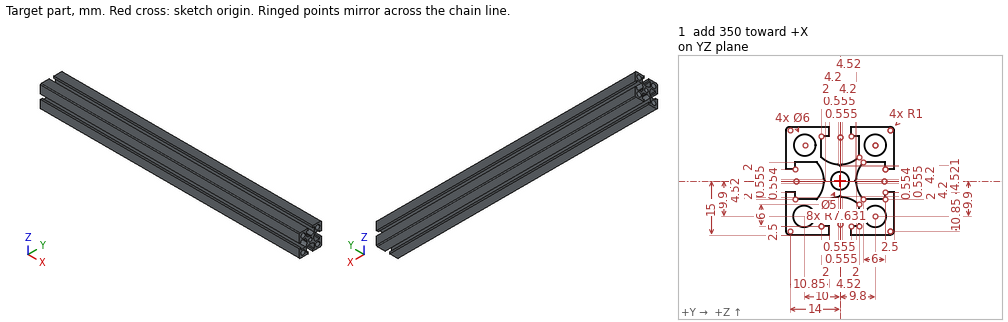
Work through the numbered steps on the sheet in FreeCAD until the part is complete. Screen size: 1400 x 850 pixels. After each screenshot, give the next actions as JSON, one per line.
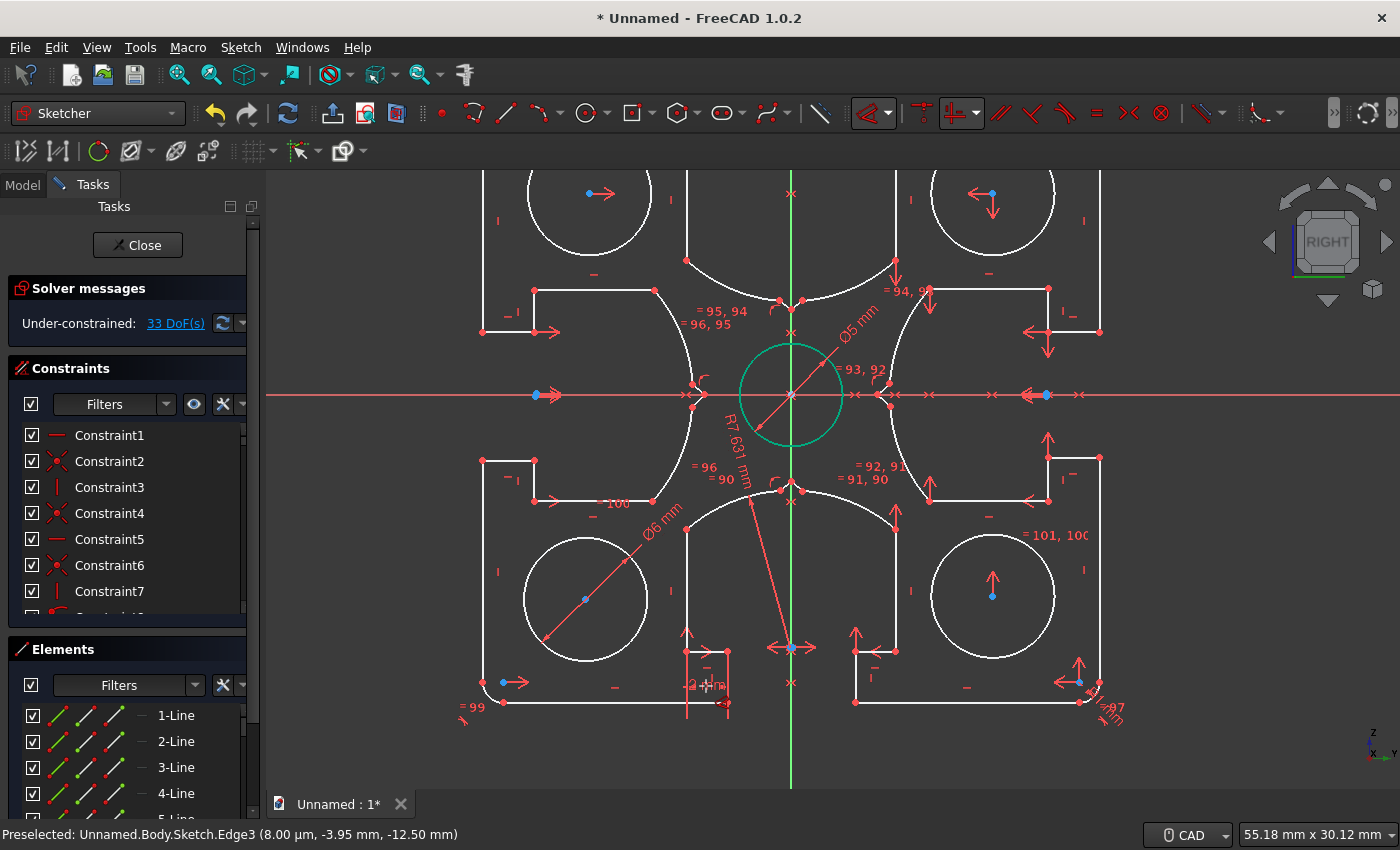
{"action": "left_click", "coordinate": [687, 615]}
{"action": "left_click", "coordinate": [653, 563]}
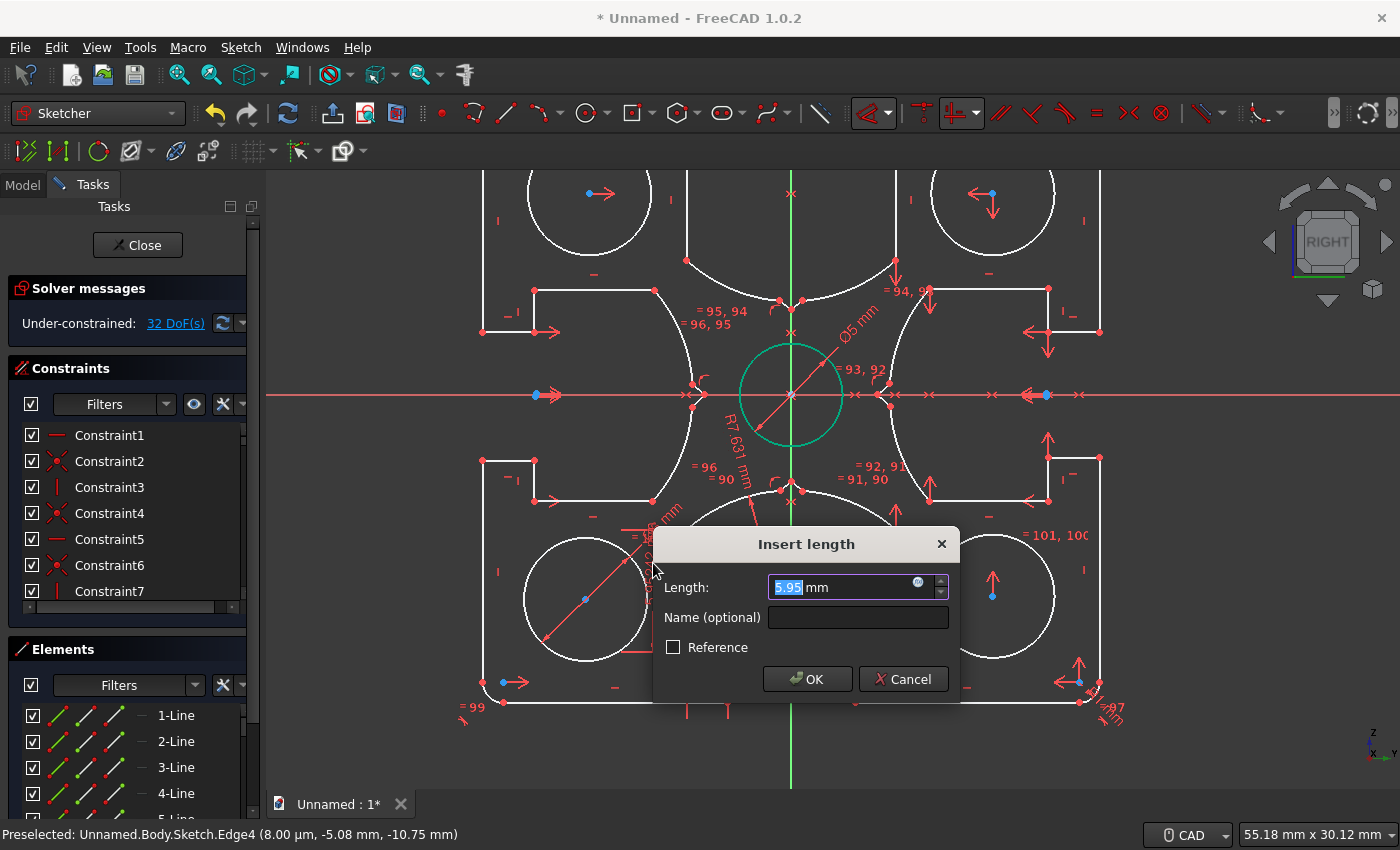
{"action": "type", "text": "6"}
{"action": "key", "text": "Return"}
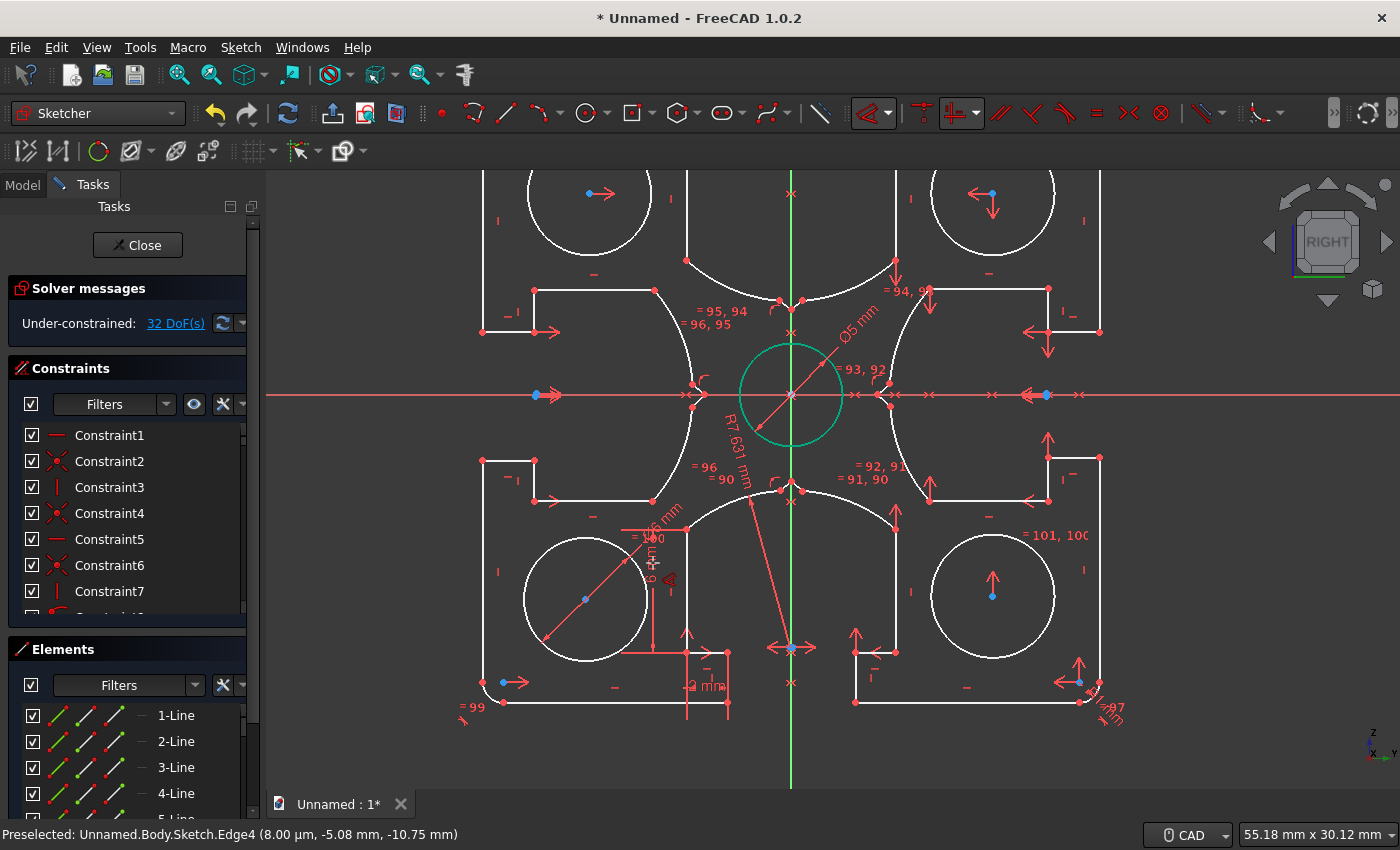
{"action": "left_click", "coordinate": [884, 653]}
{"action": "left_click", "coordinate": [876, 687]}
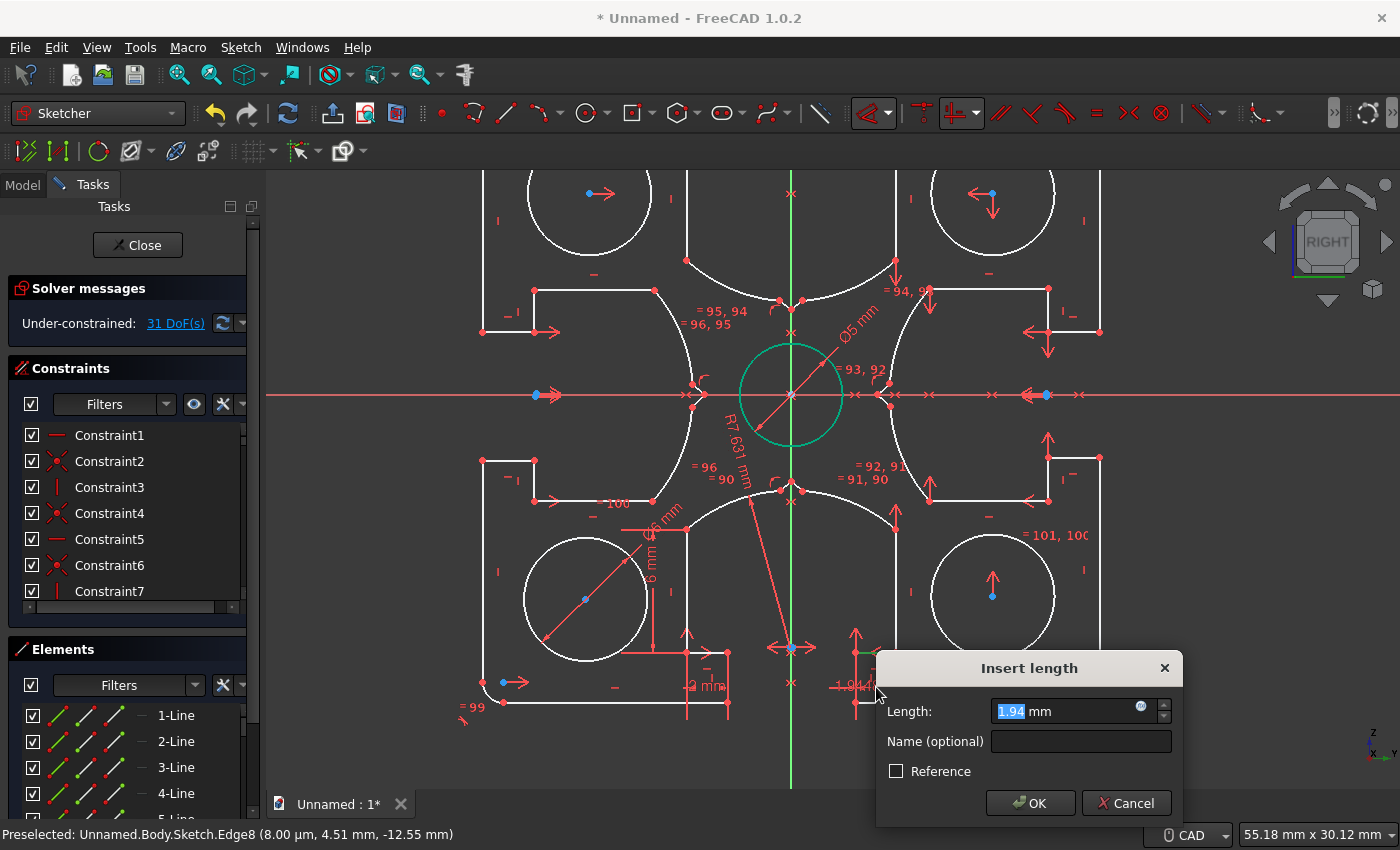
{"action": "type", "text": "2"}
{"action": "key", "text": "Return"}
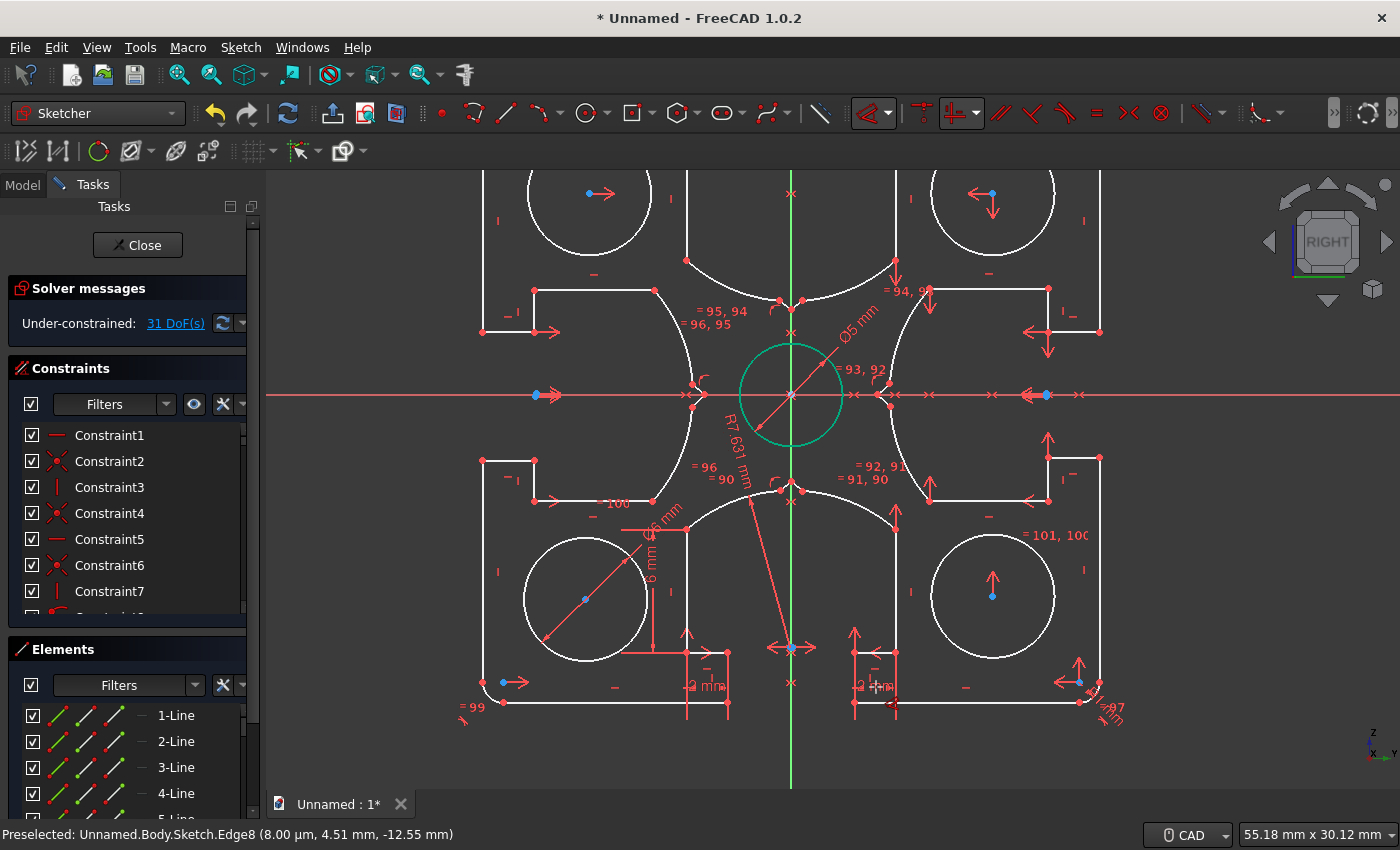
{"action": "left_click", "coordinate": [1048, 471]}
{"action": "left_click", "coordinate": [1082, 479]}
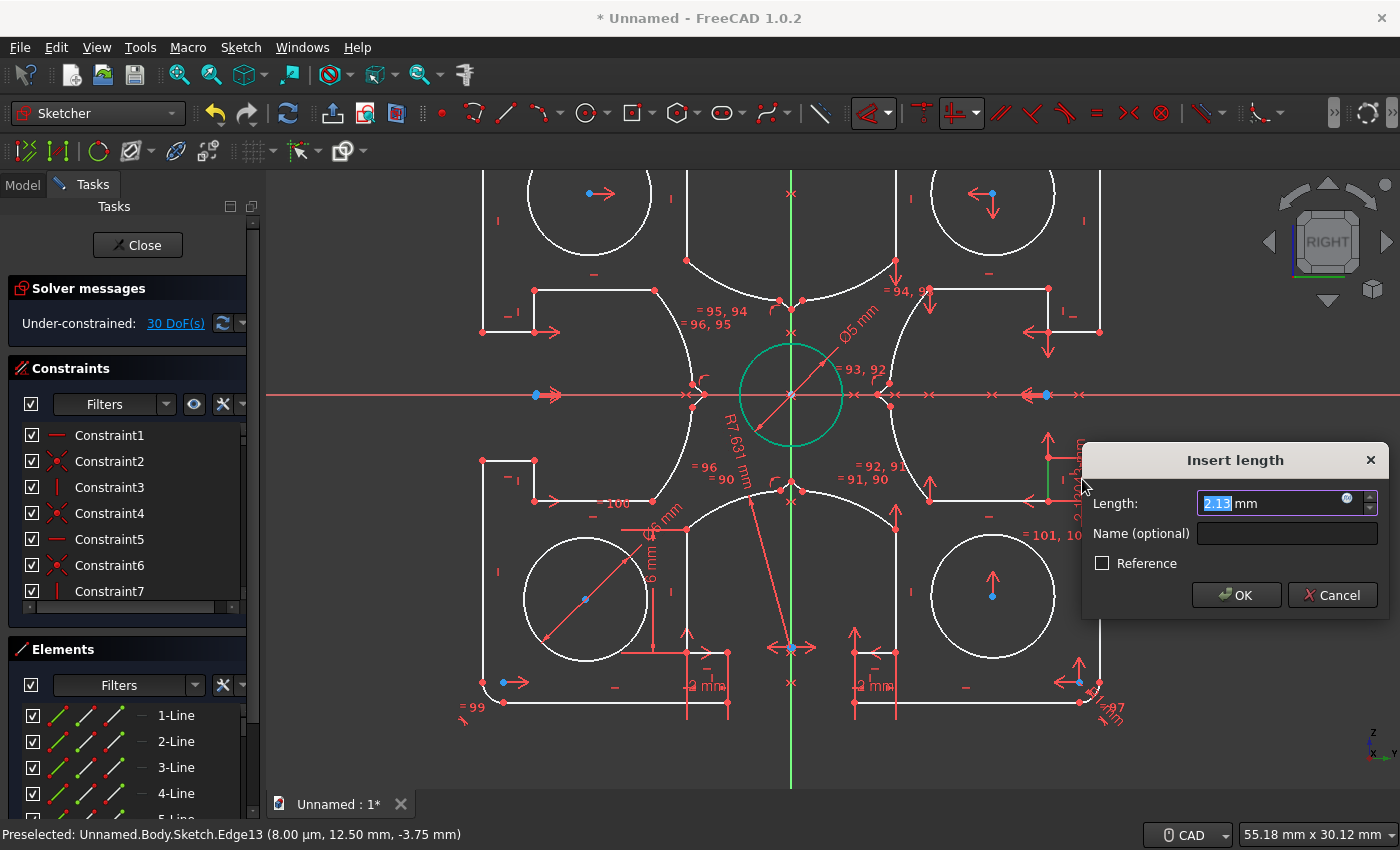
{"action": "type", "text": "2"}
{"action": "key", "text": "Return"}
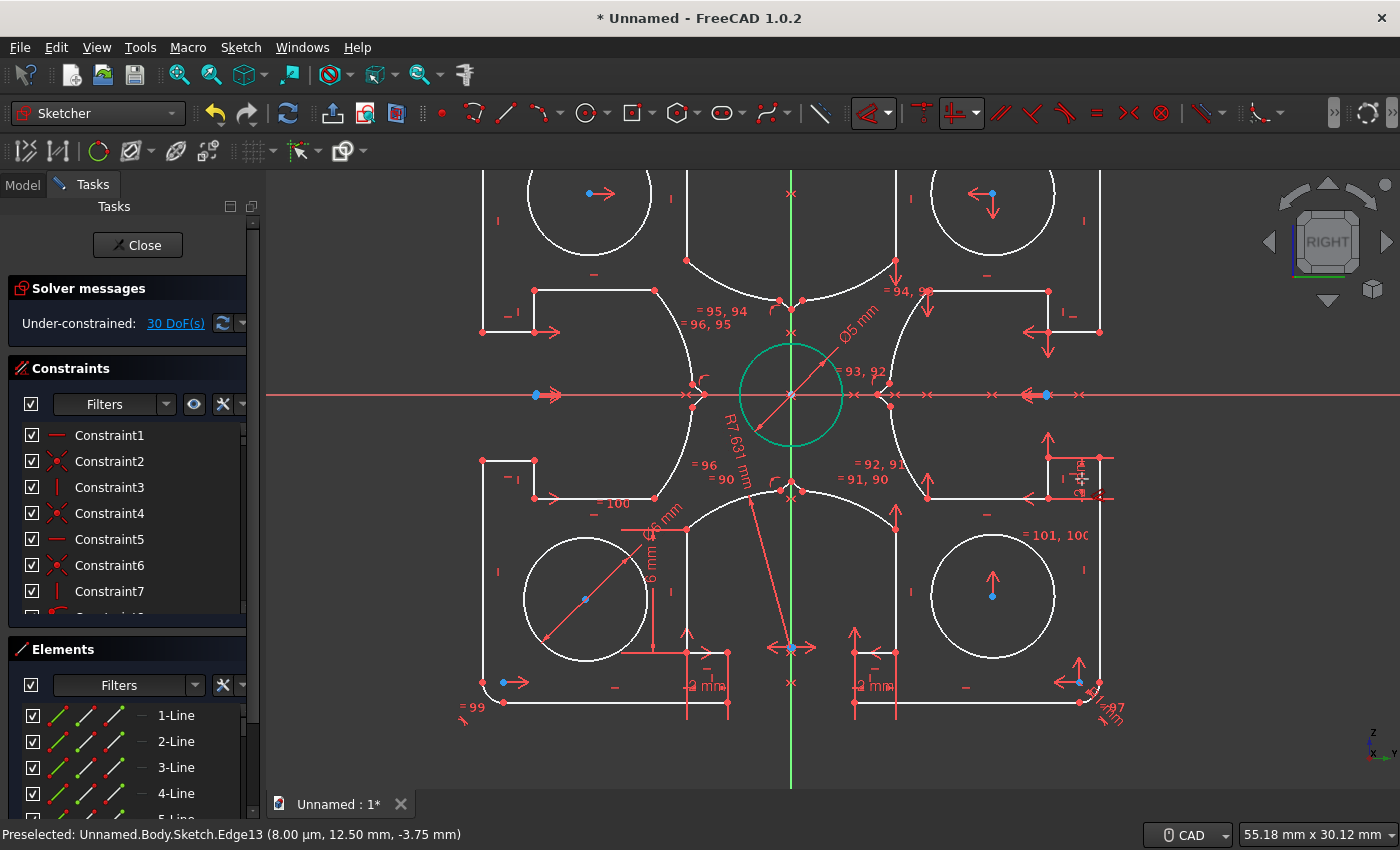
{"action": "left_click", "coordinate": [1012, 499]}
{"action": "left_click", "coordinate": [946, 533]}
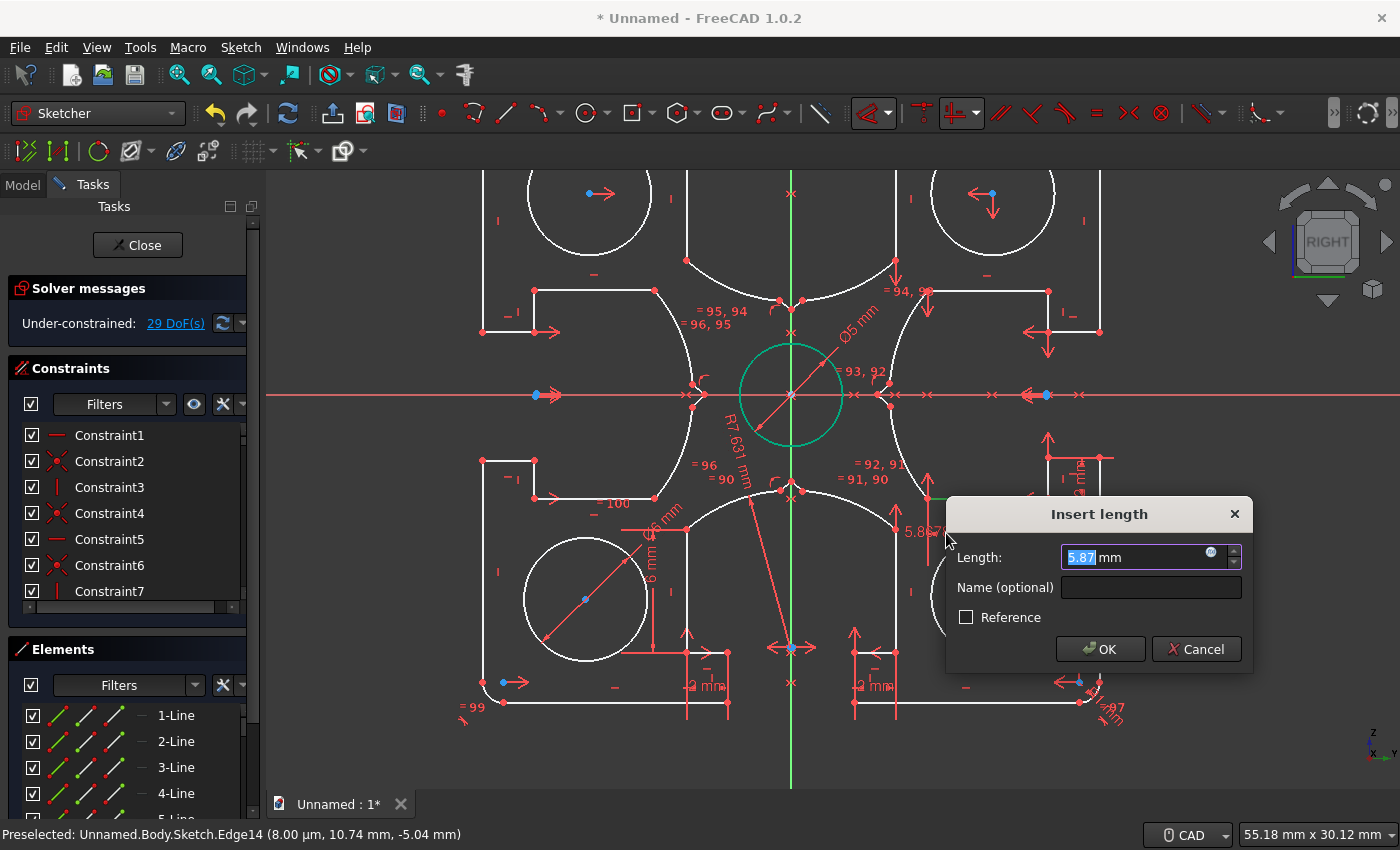
{"action": "type", "text": "6"}
{"action": "key", "text": "Return"}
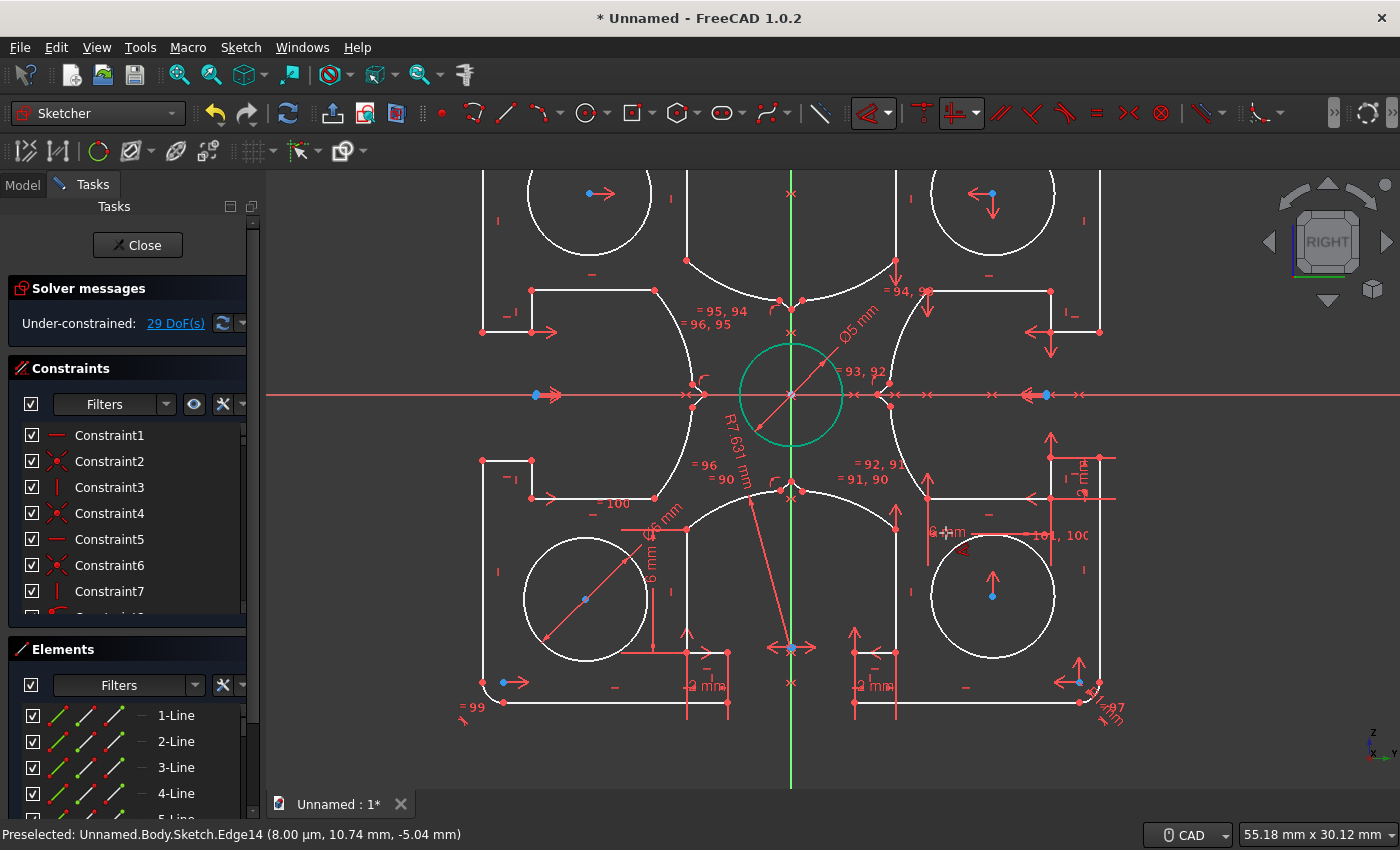
{"action": "scroll", "coordinate": [710, 651], "scroll_direction": "down", "scroll_amount": 2}